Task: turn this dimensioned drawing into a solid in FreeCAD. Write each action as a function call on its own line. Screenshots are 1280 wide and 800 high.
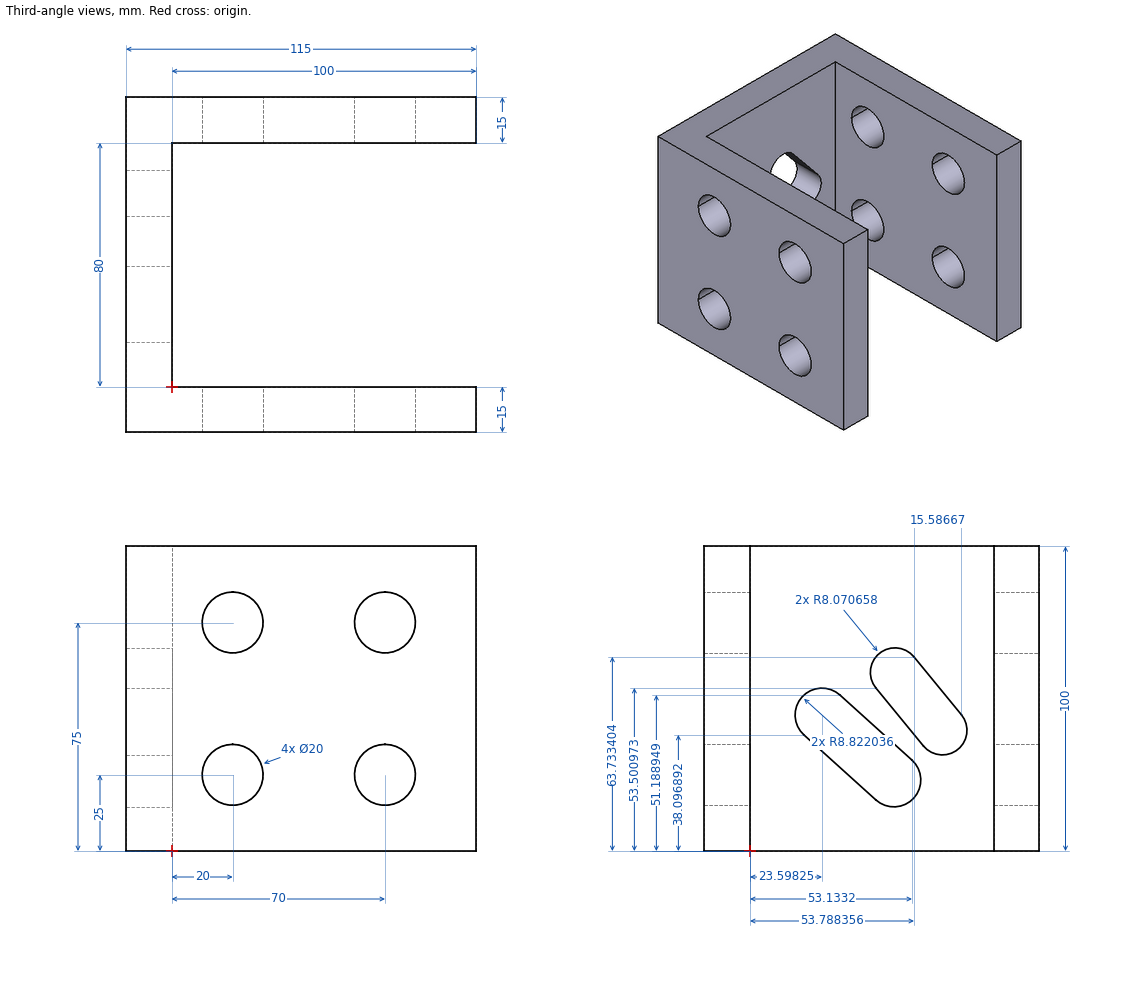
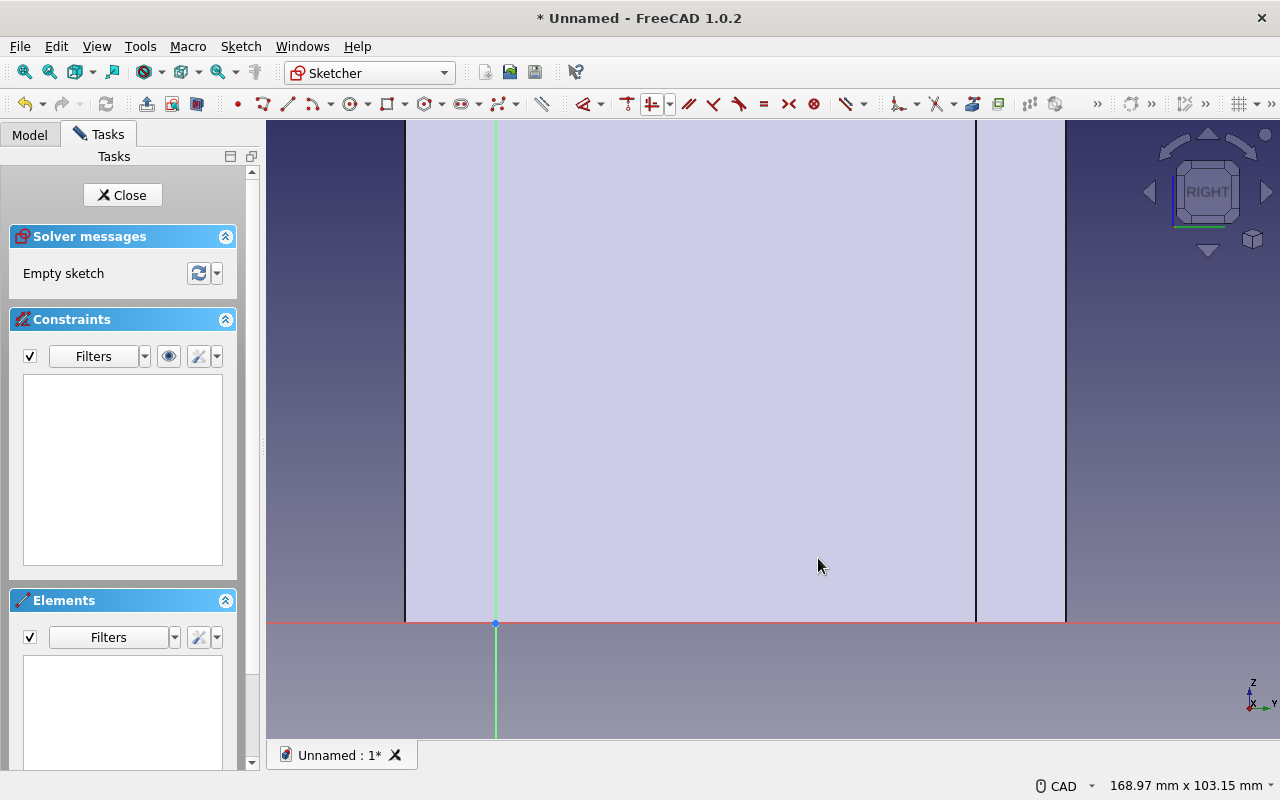
click(460, 104)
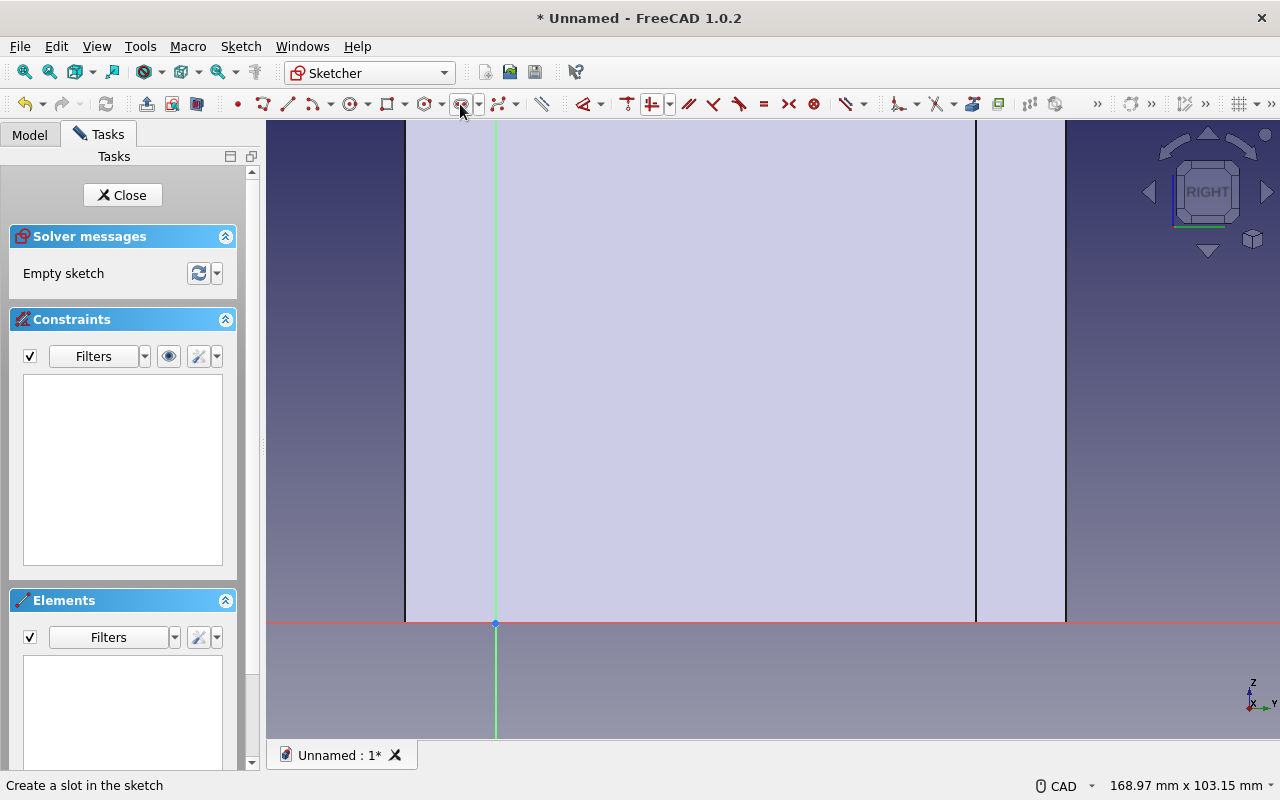
click(781, 272)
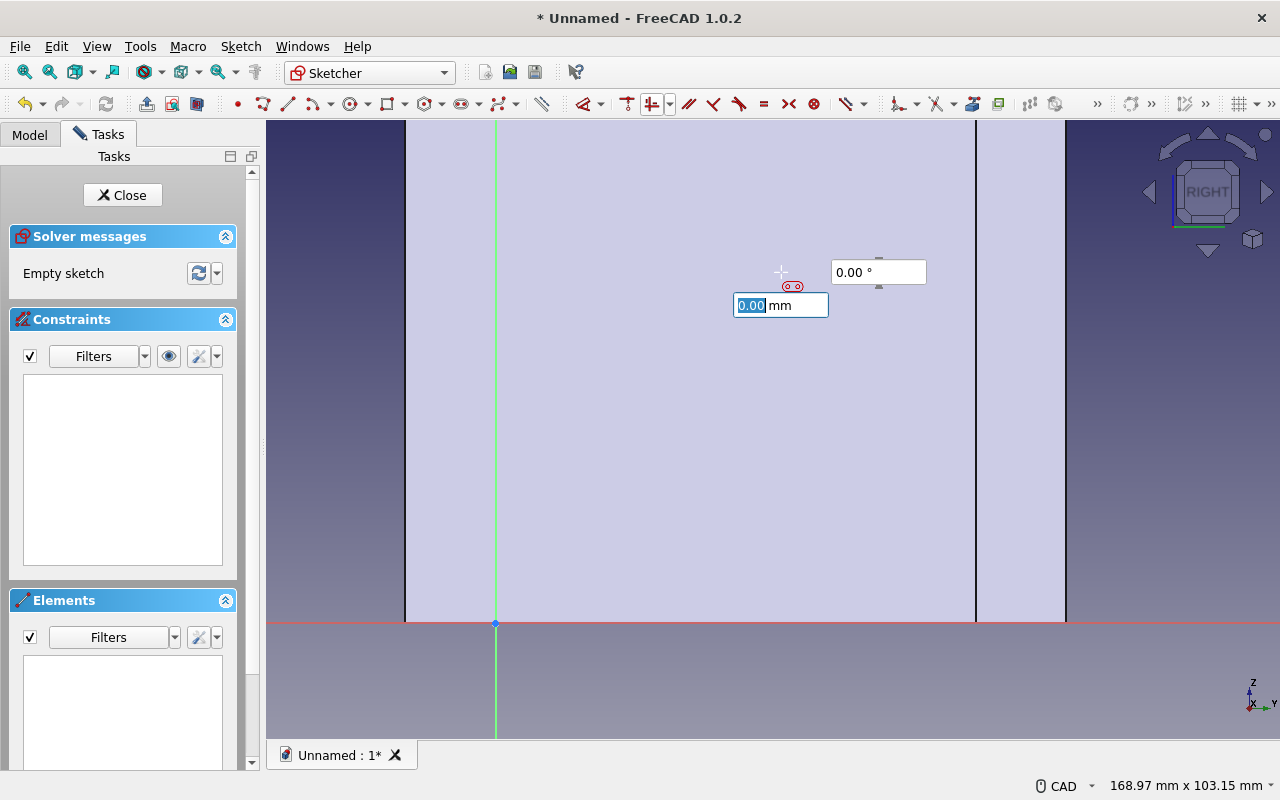
click(874, 386)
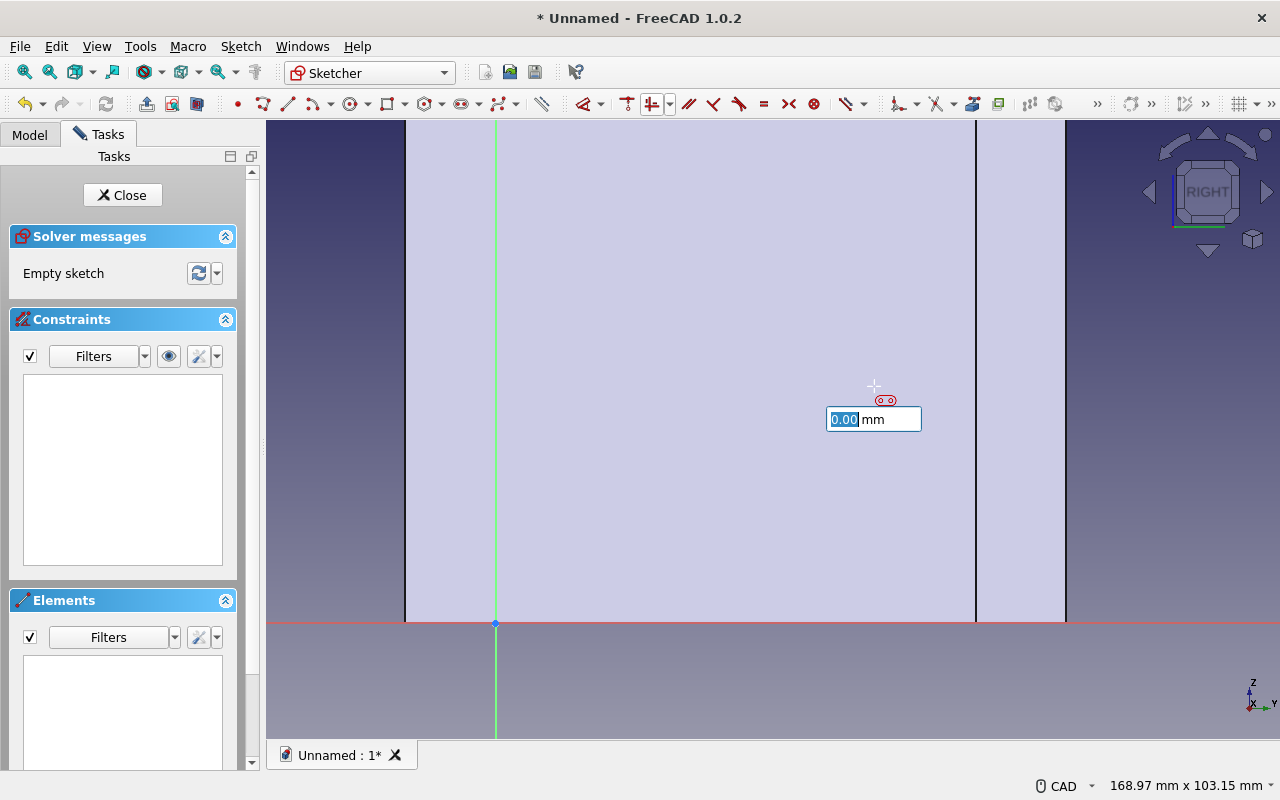
click(865, 298)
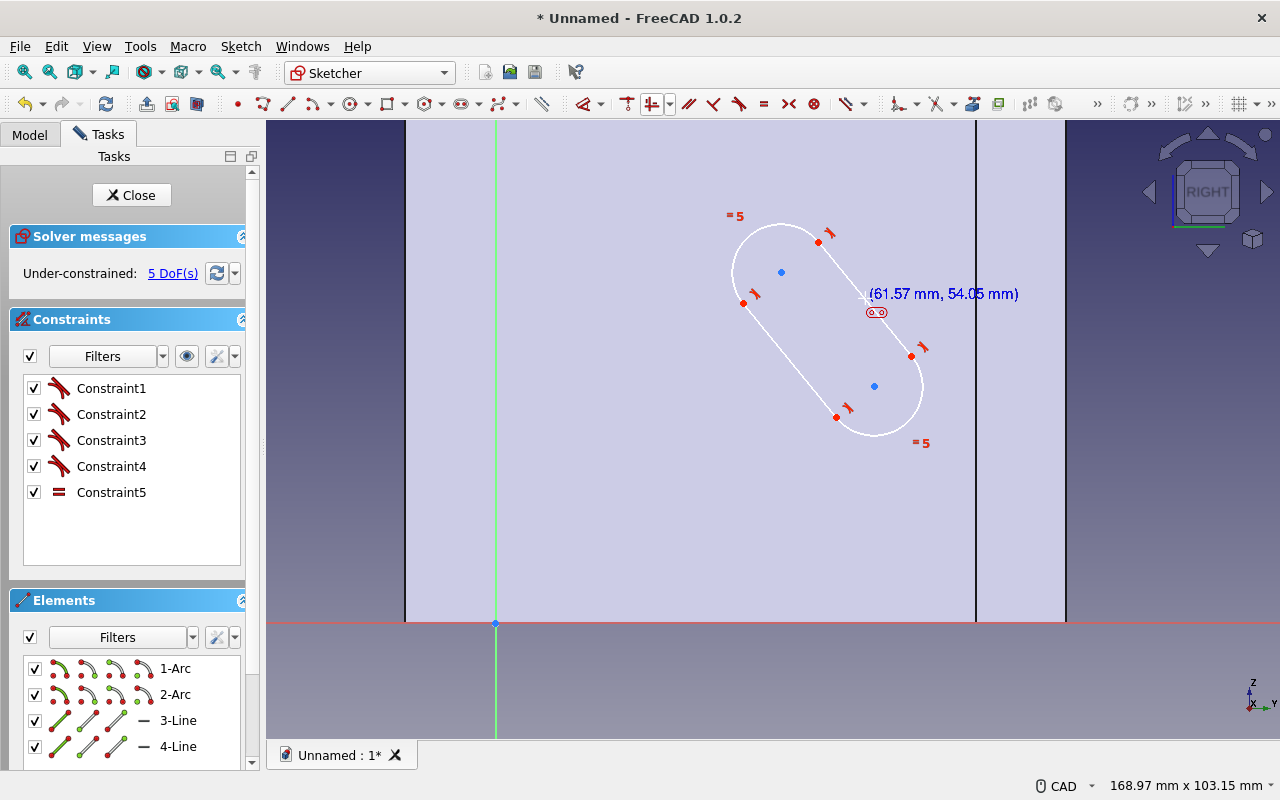
click(637, 355)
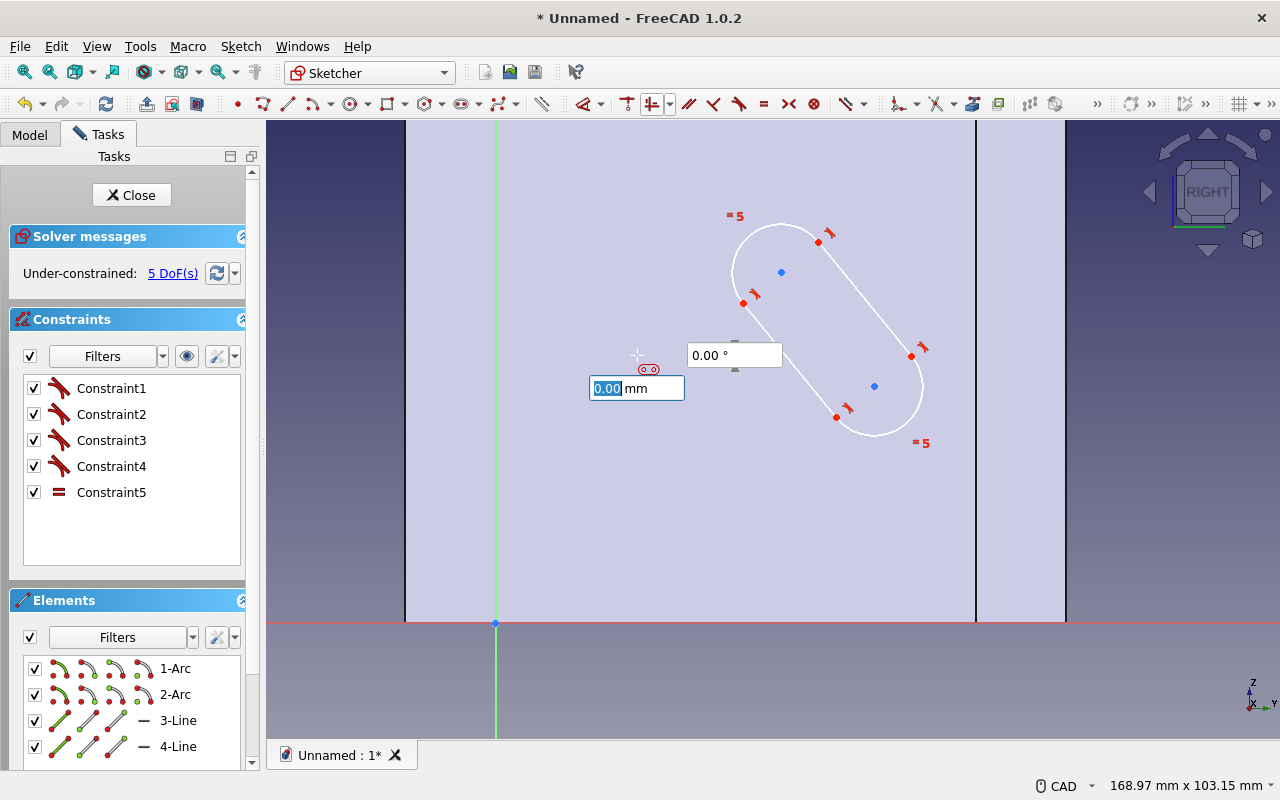
click(779, 483)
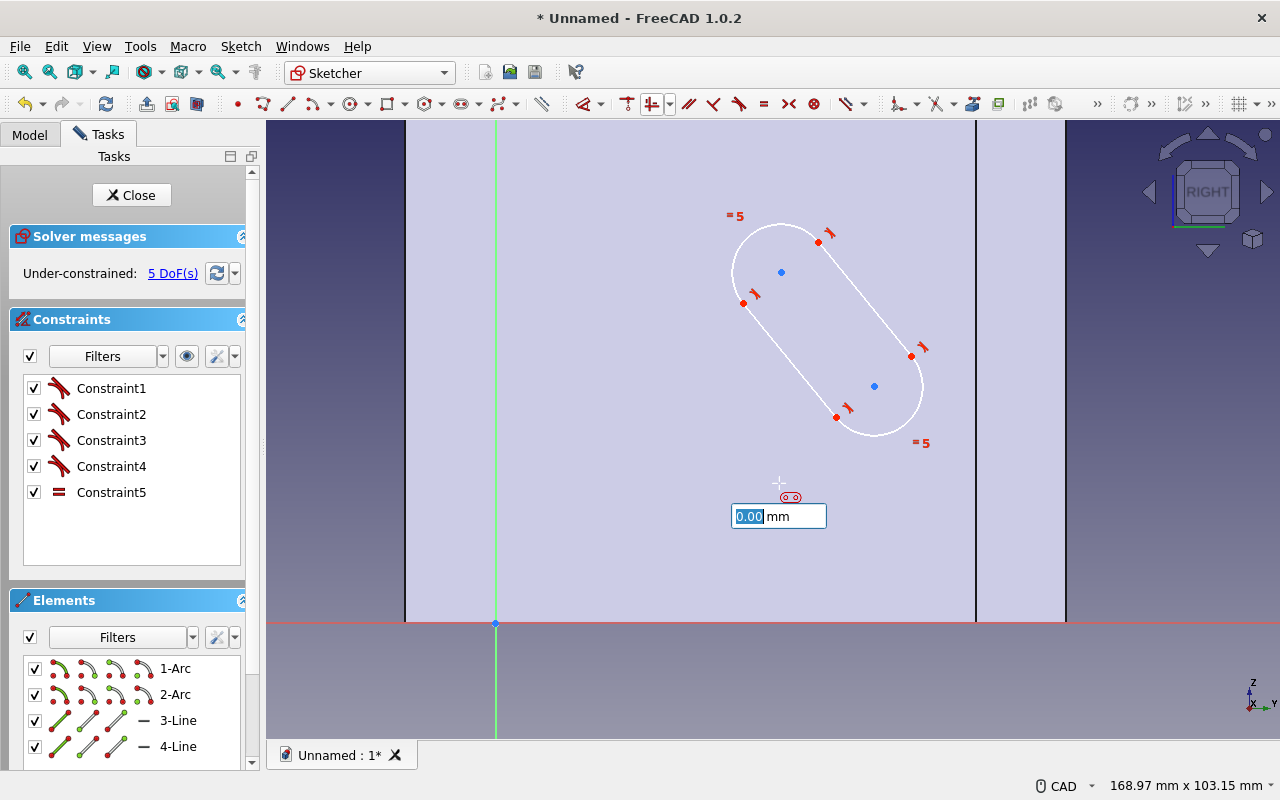
click(743, 380)
key(Escape)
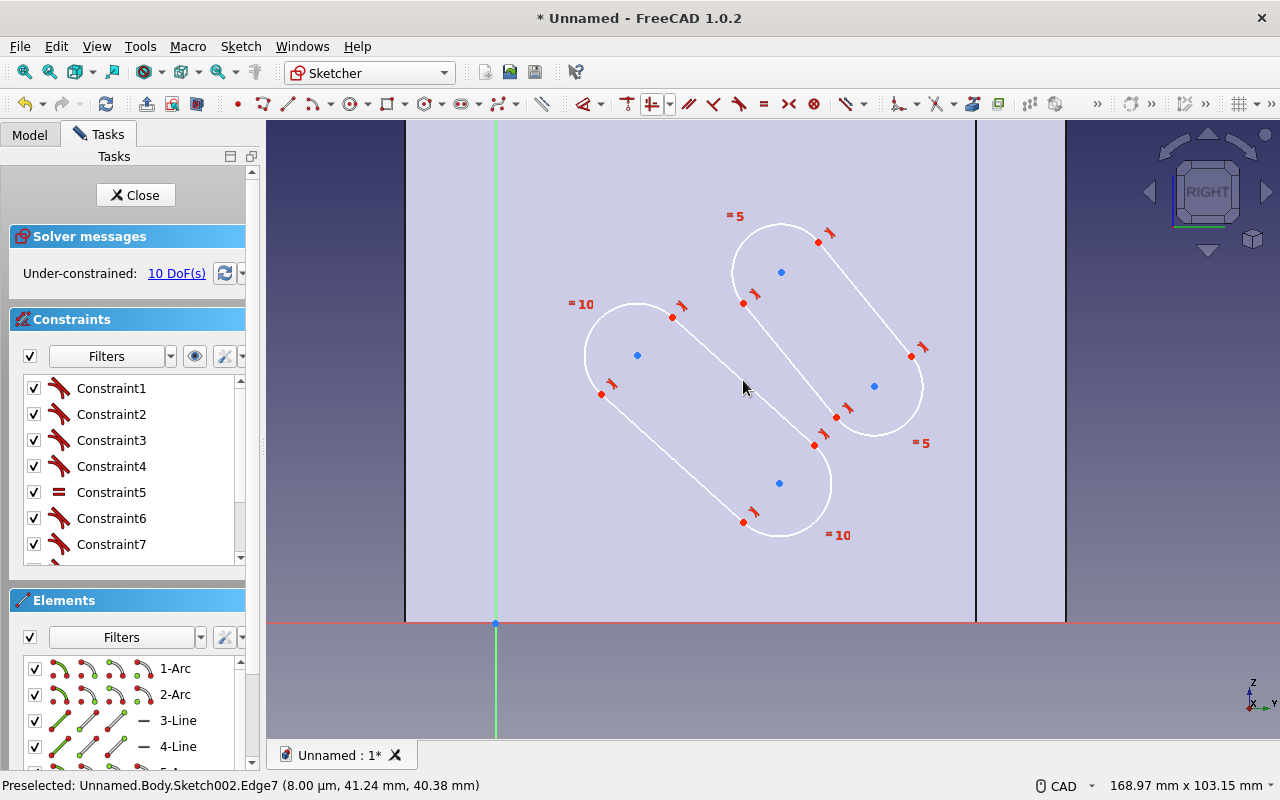
click(582, 104)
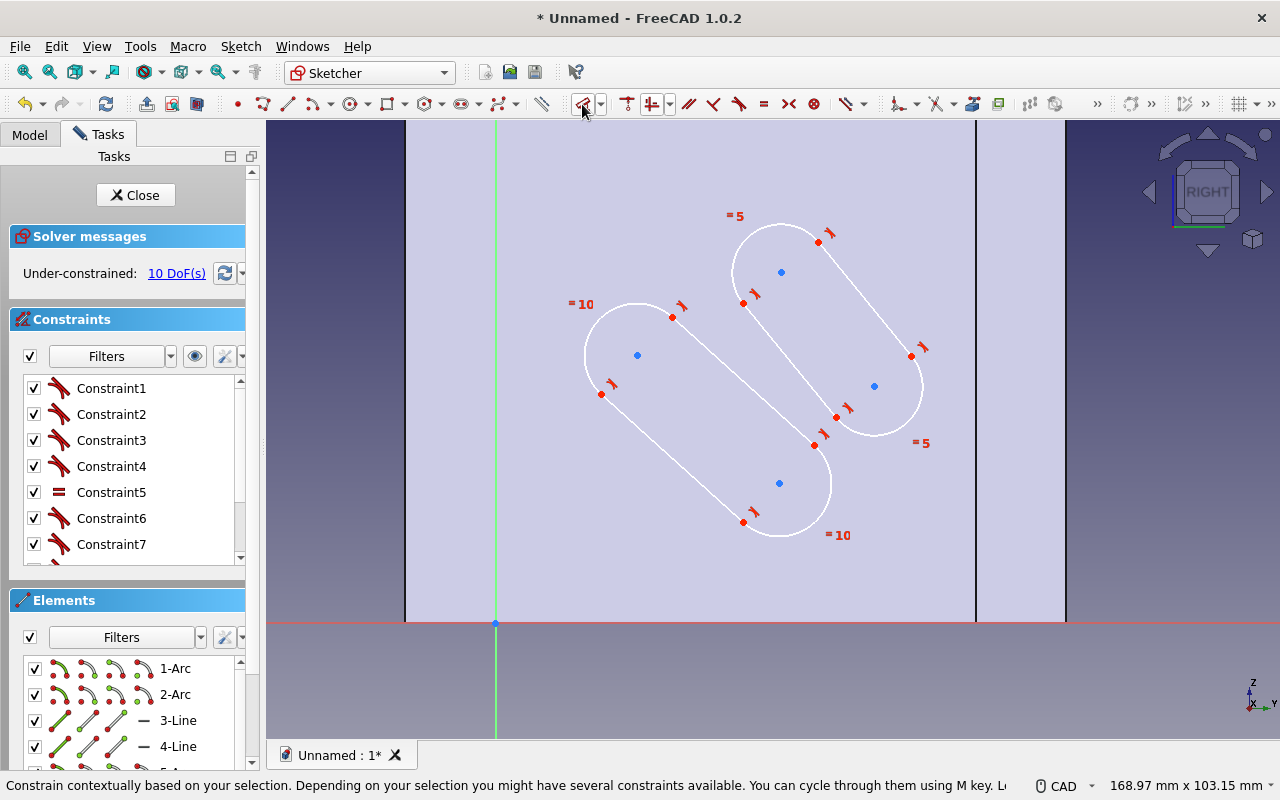
click(778, 224)
click(776, 192)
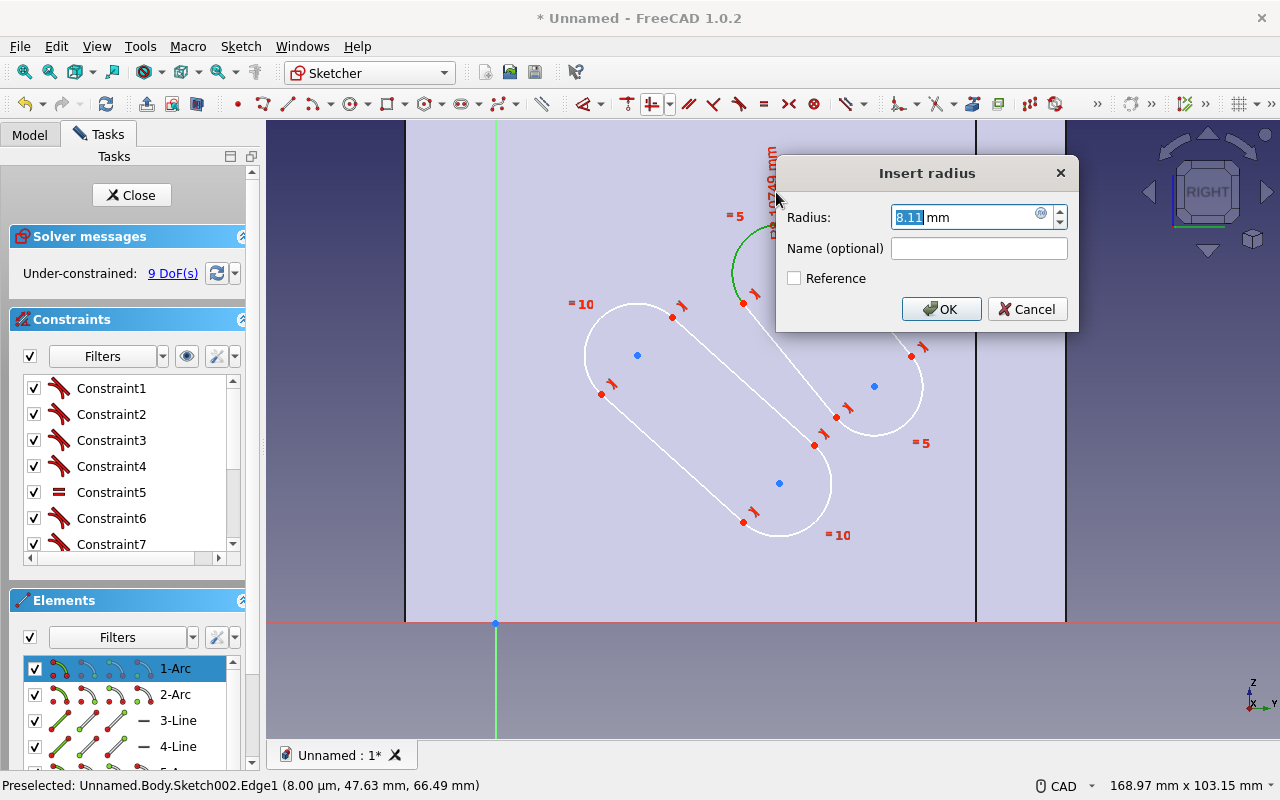
text(8.070658)
key(Return)